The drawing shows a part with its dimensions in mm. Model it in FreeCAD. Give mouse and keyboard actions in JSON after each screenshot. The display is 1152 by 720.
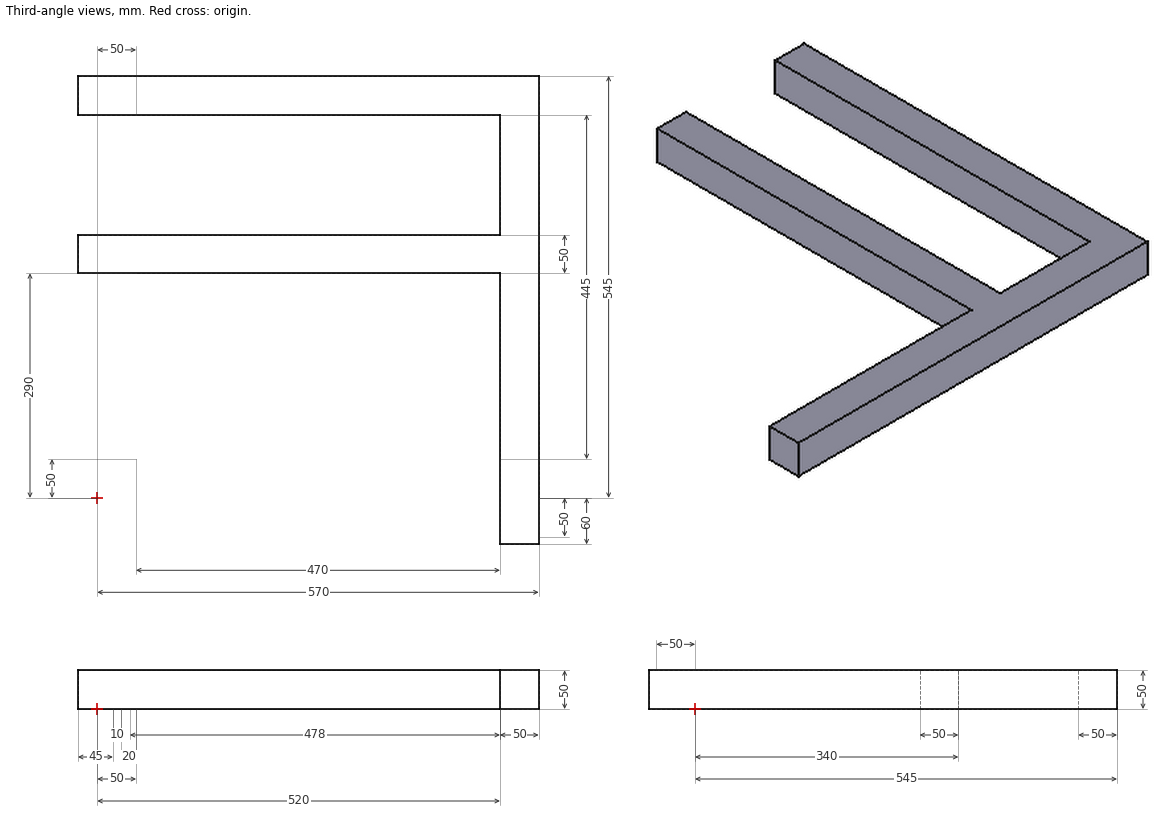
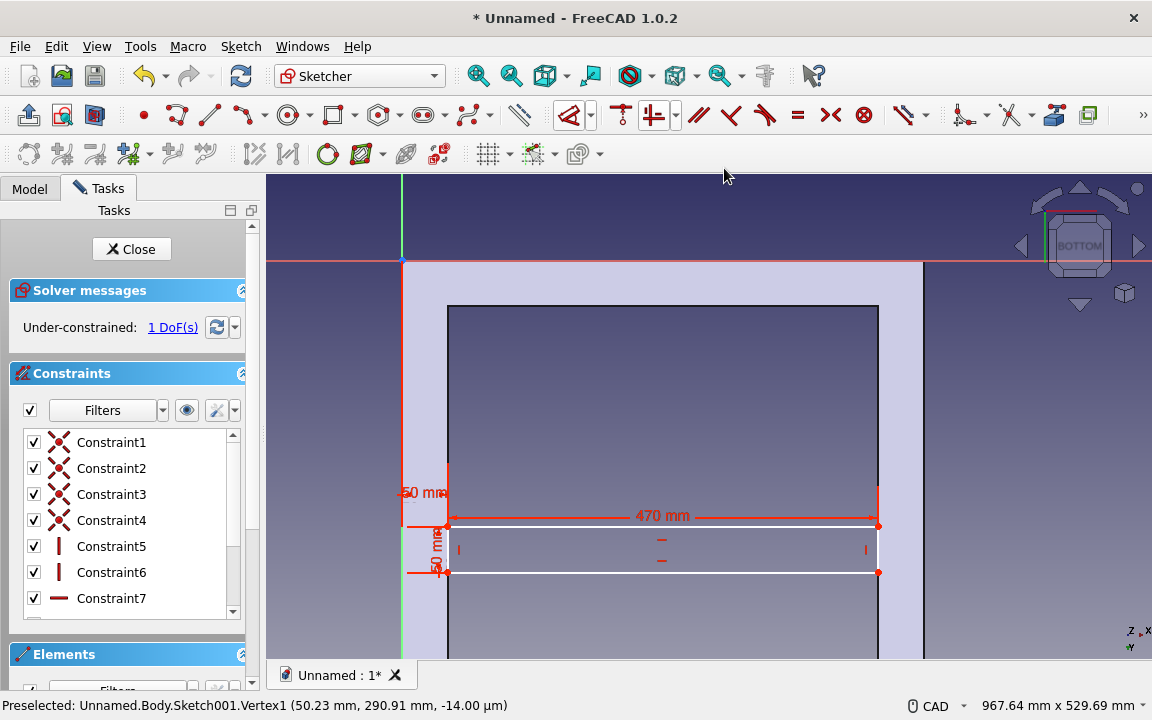
{"action": "left_click", "coordinate": [448, 527]}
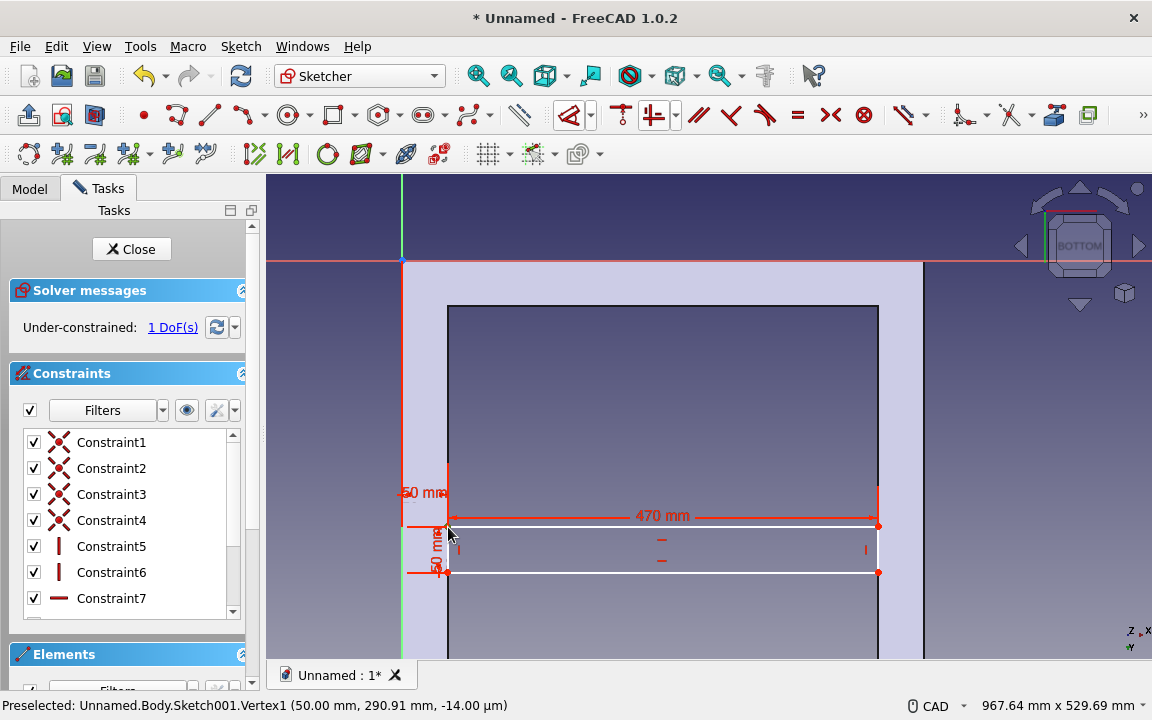
{"action": "key", "text": "i"}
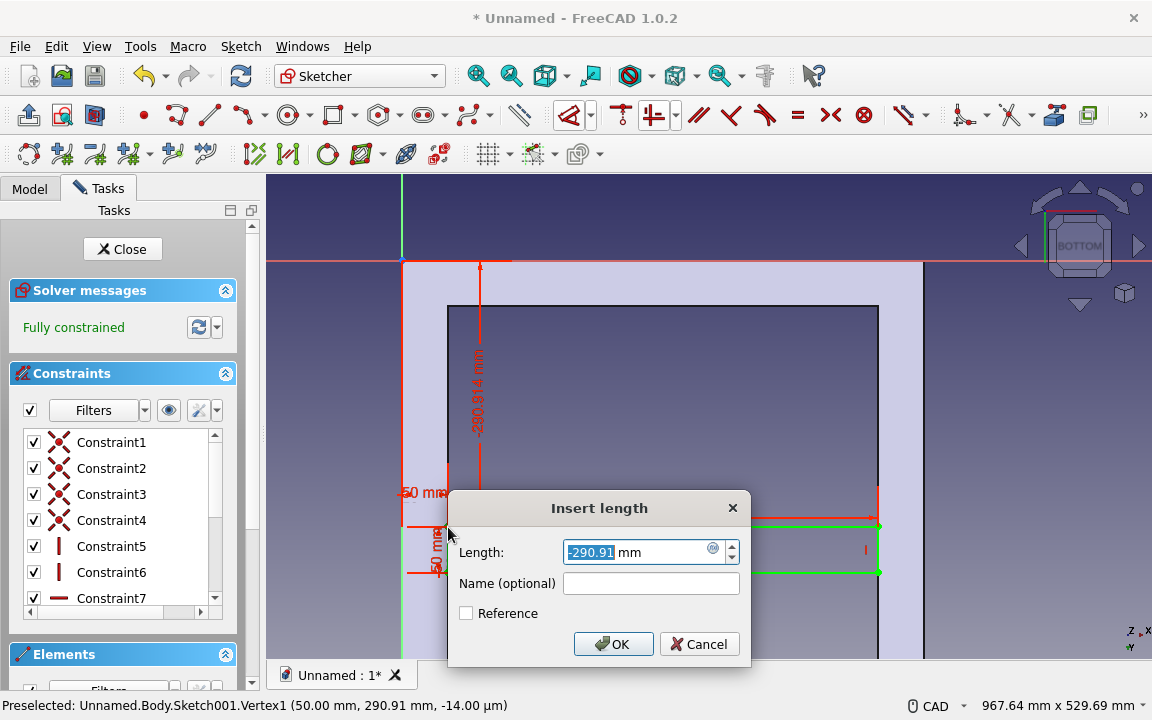
{"action": "type", "text": "-290"}
{"action": "key", "text": "Return"}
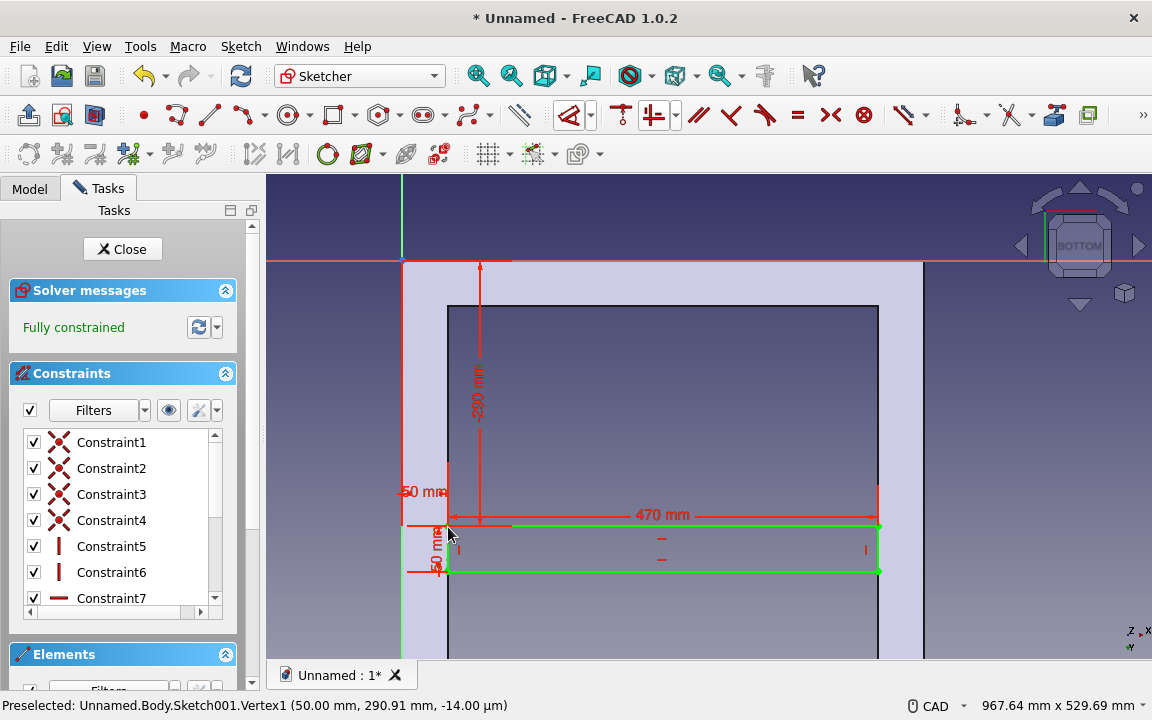
{"action": "left_click", "coordinate": [123, 249]}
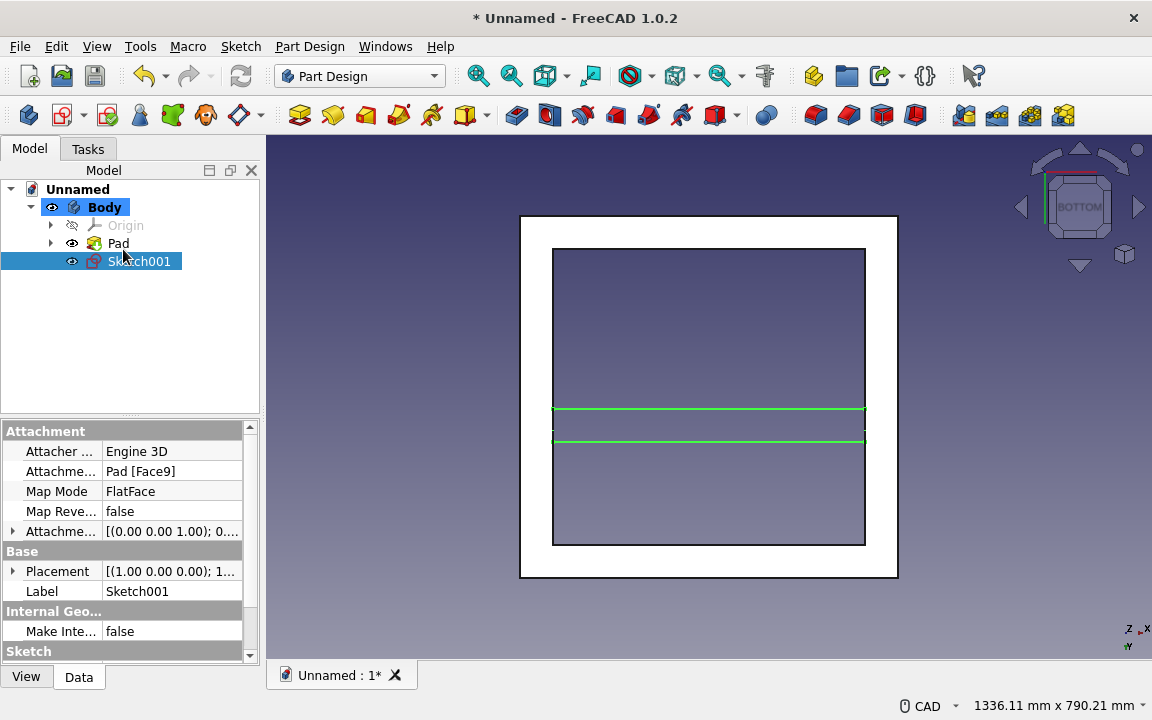
{"action": "left_click", "coordinate": [300, 116]}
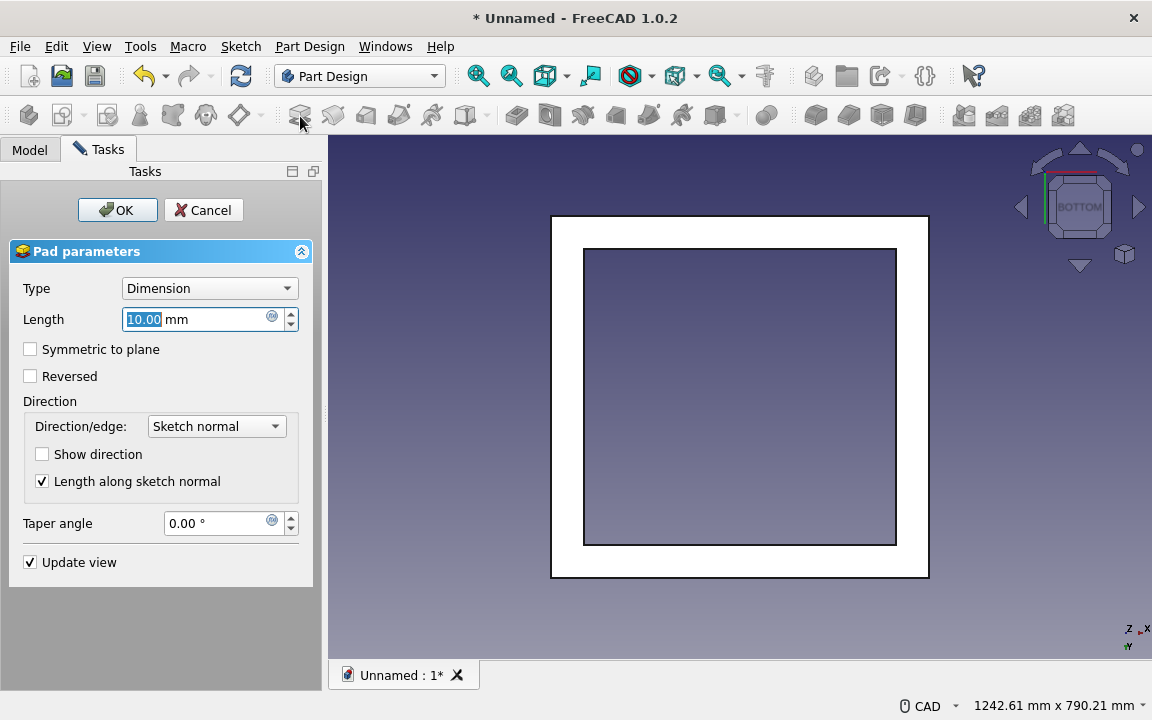
{"action": "type", "text": "50"}
{"action": "key", "text": "Tab"}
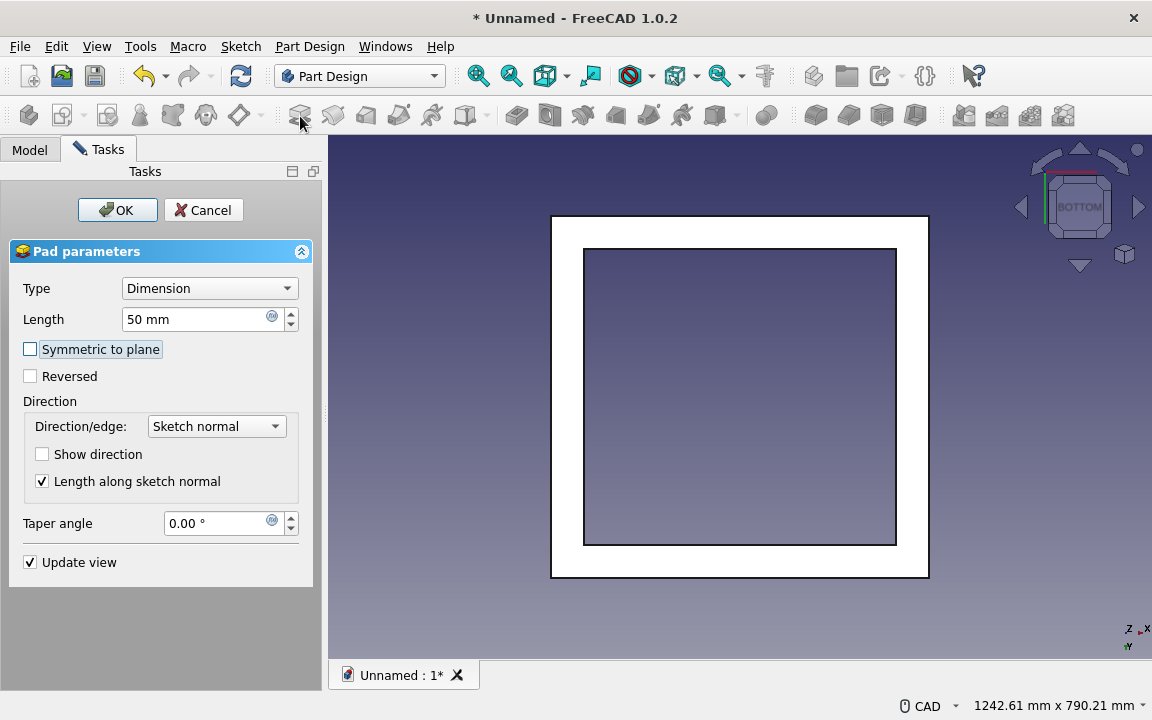
{"action": "left_click", "coordinate": [31, 376]}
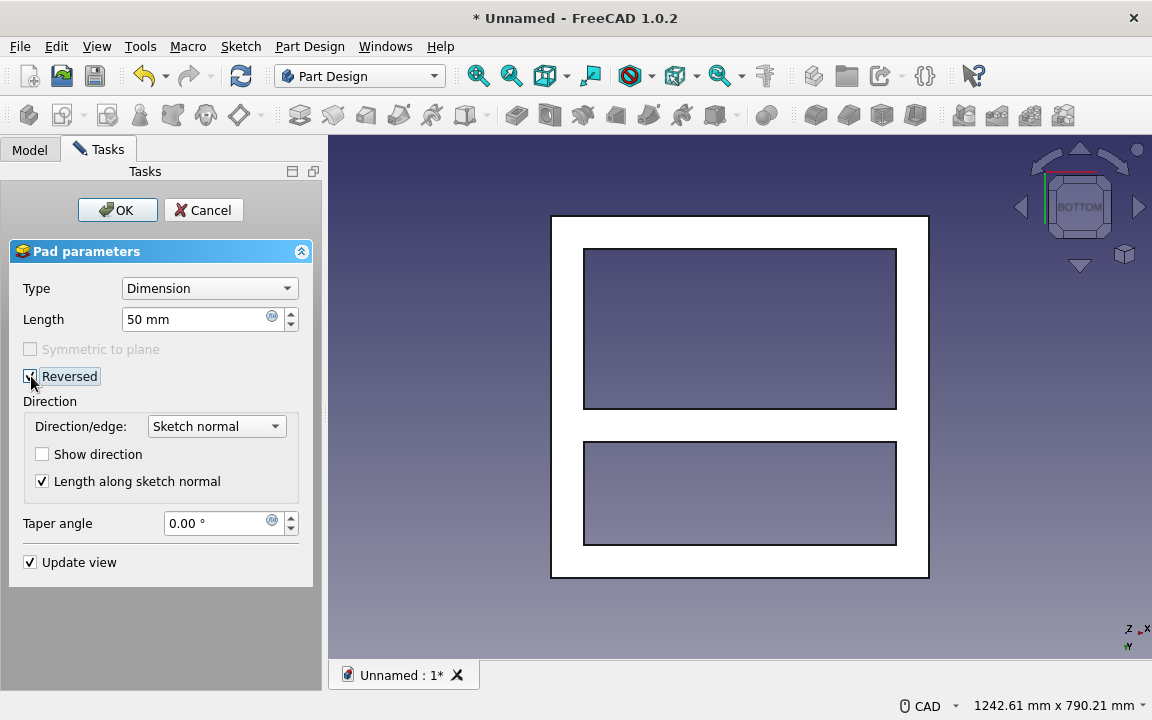
{"action": "left_click", "coordinate": [118, 210]}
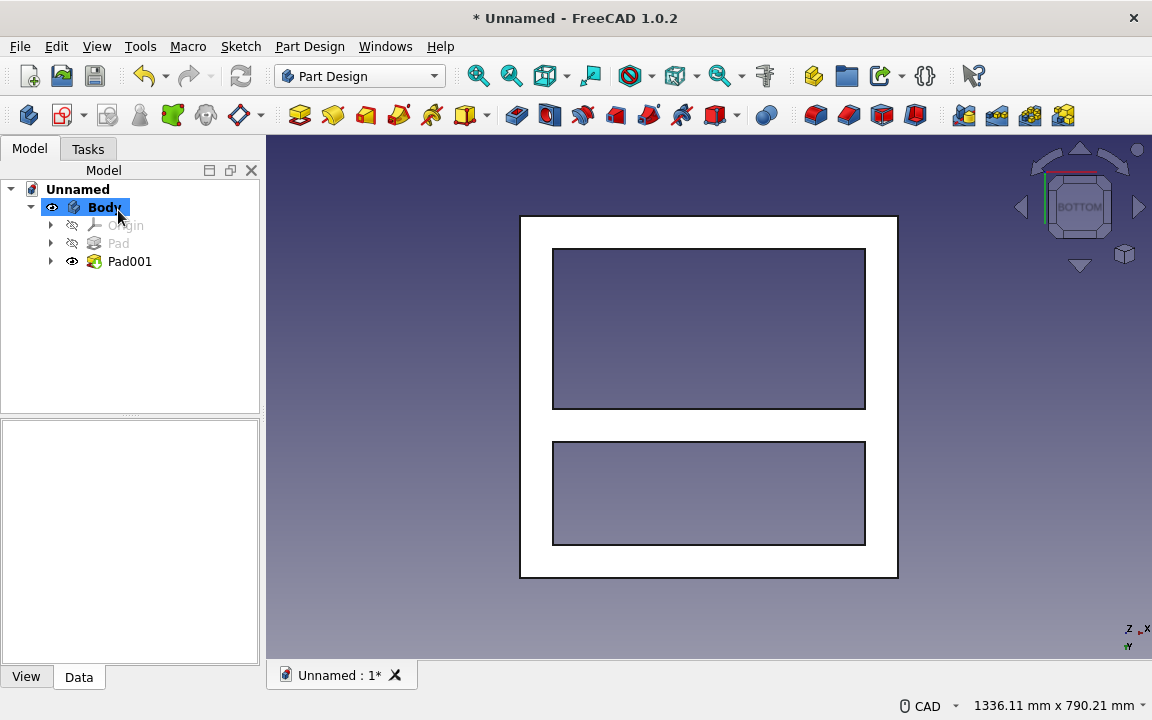
{"action": "left_click", "coordinate": [62, 116]}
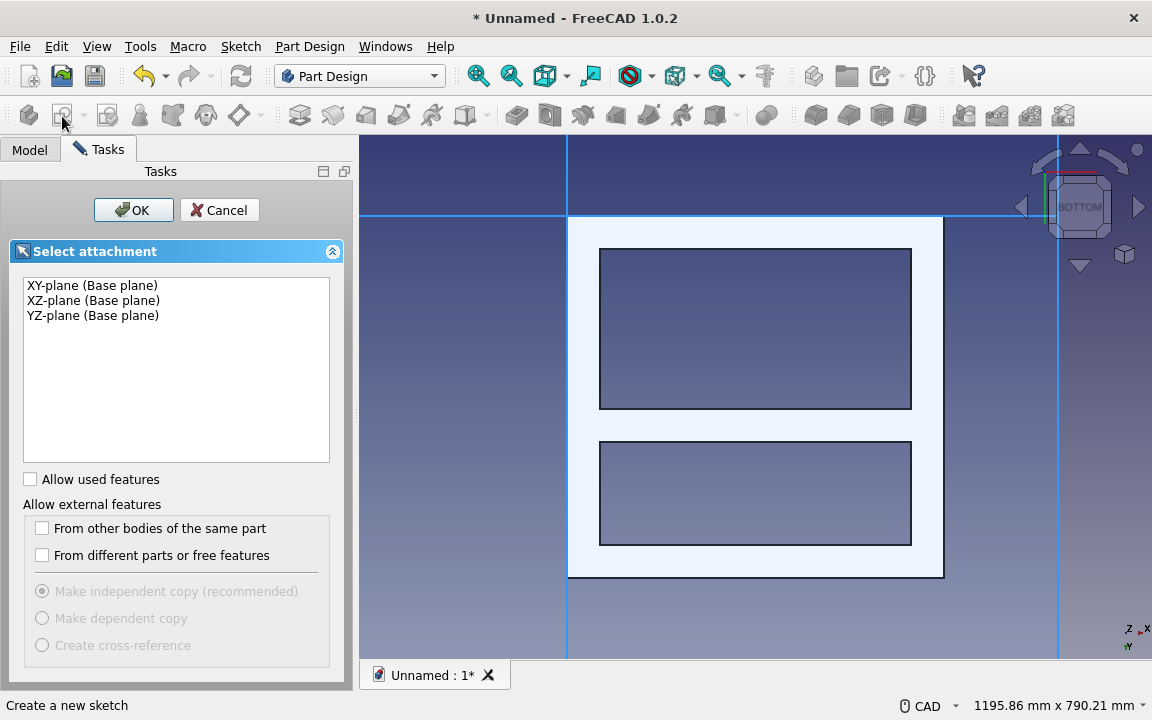
{"action": "left_click", "coordinate": [84, 300]}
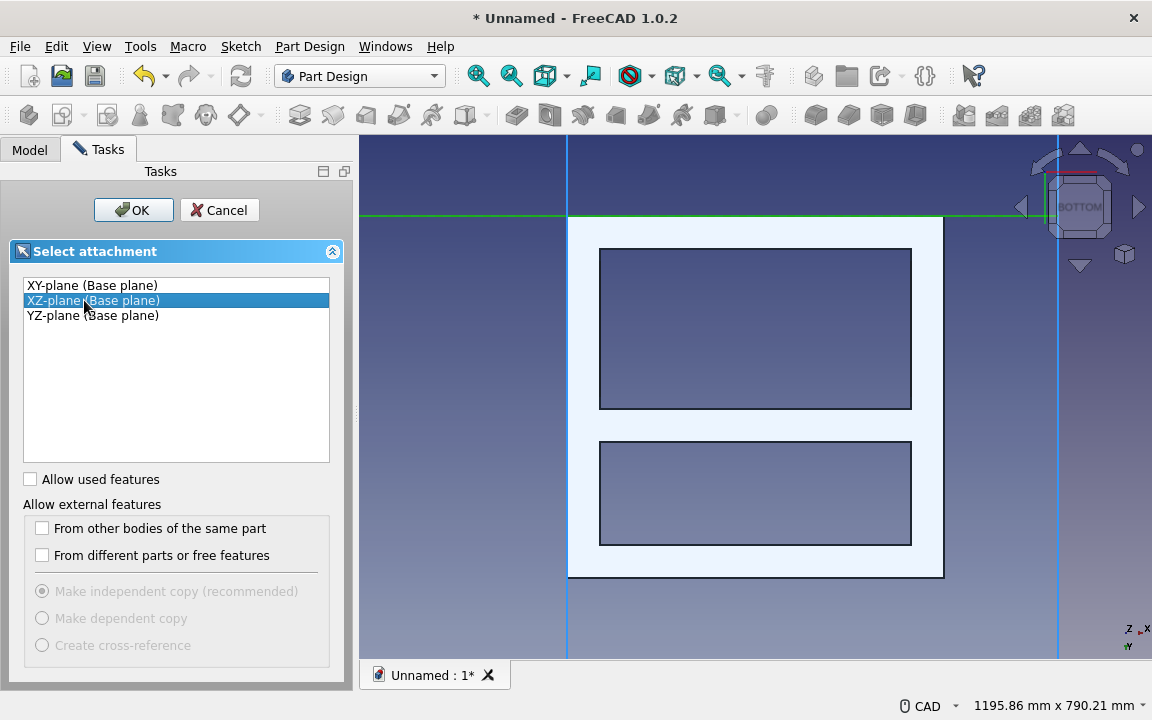
{"action": "left_click", "coordinate": [134, 210]}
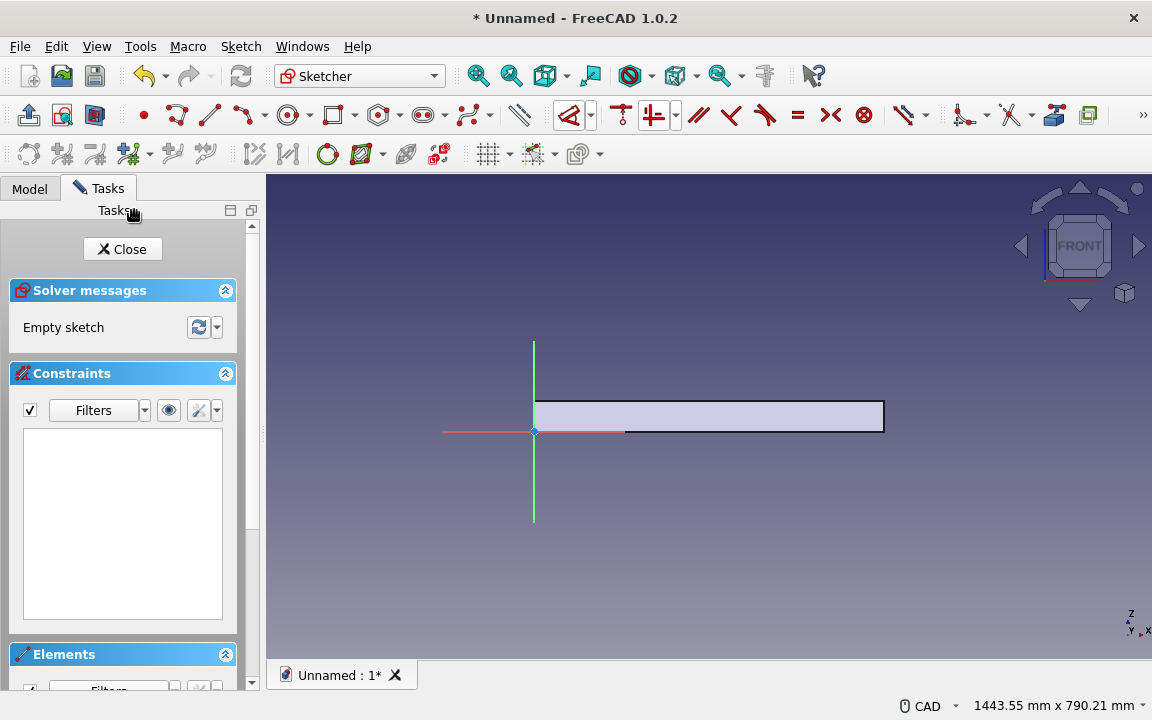
{"action": "scroll", "coordinate": [848, 417], "scroll_direction": "up", "scroll_amount": 2}